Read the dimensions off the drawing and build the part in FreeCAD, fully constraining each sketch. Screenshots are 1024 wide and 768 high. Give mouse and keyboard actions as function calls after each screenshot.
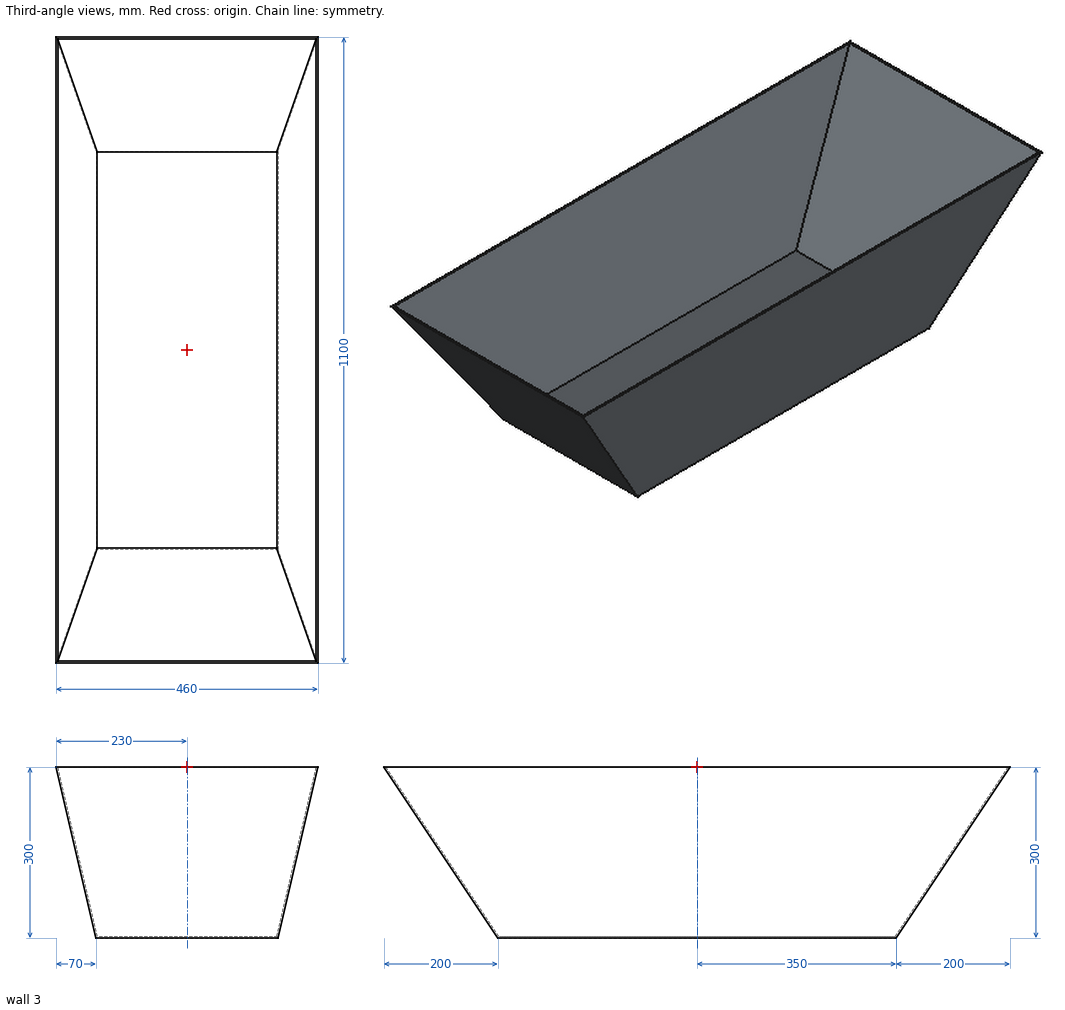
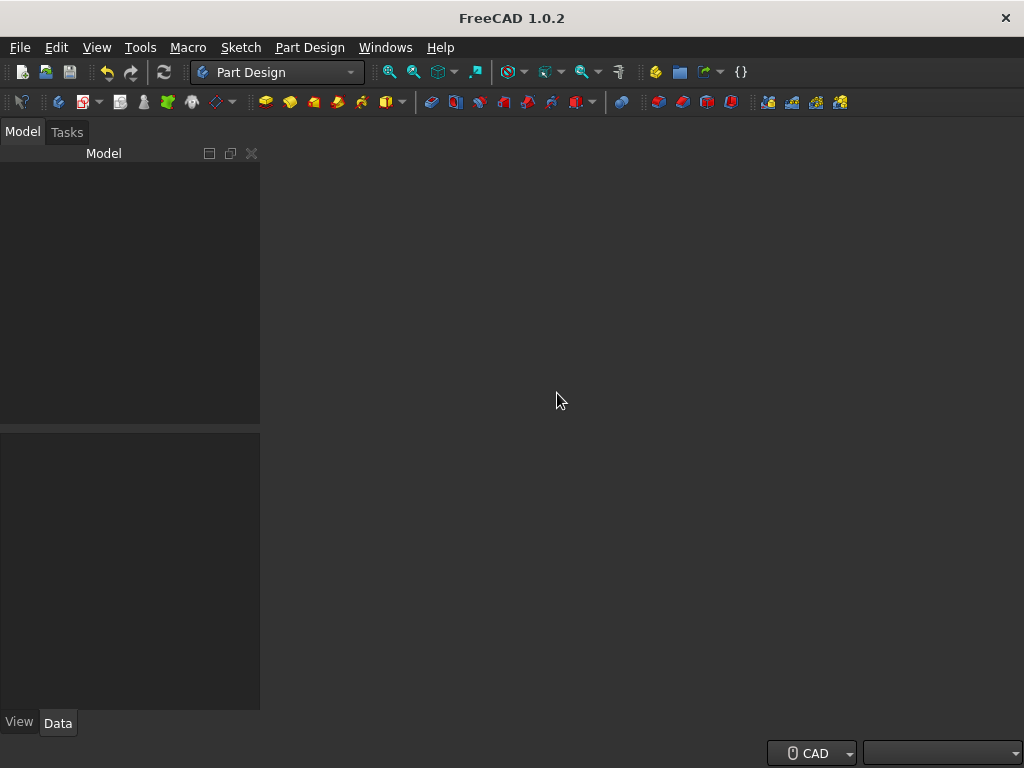
click(22, 72)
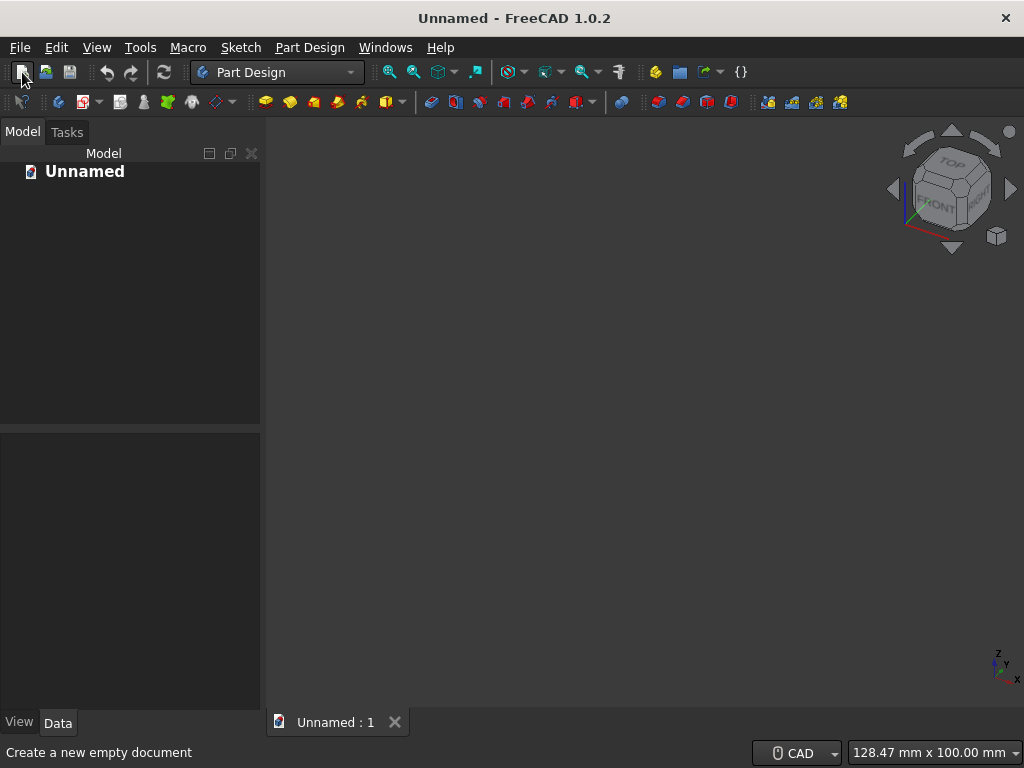
click(84, 102)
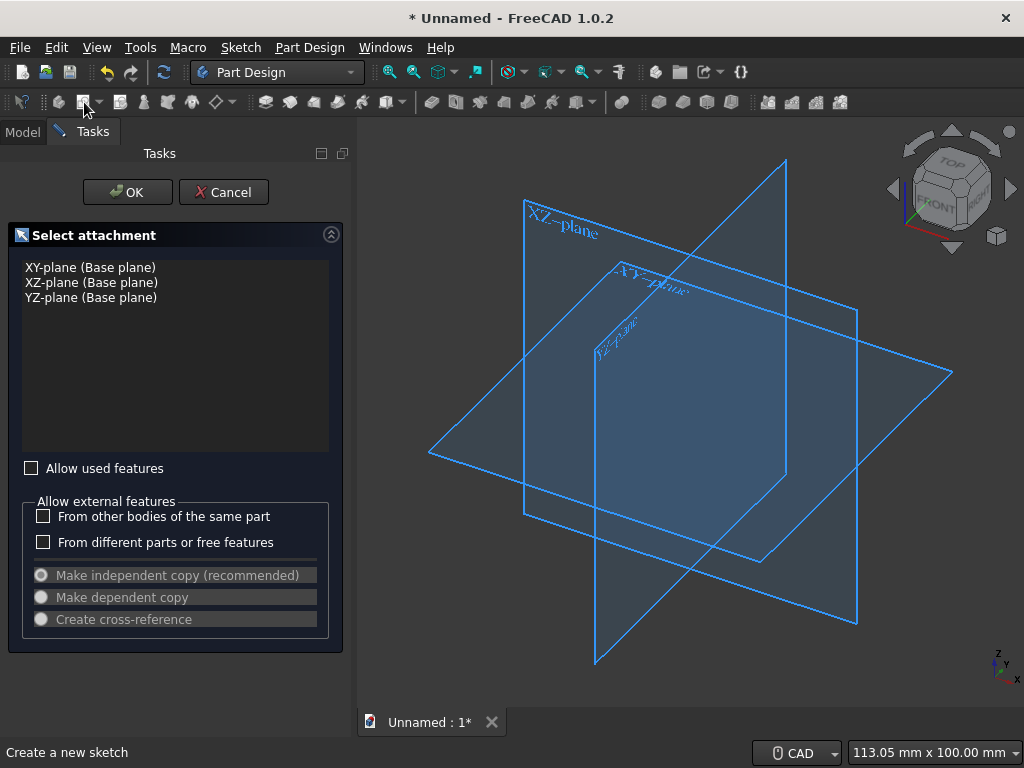
click(82, 268)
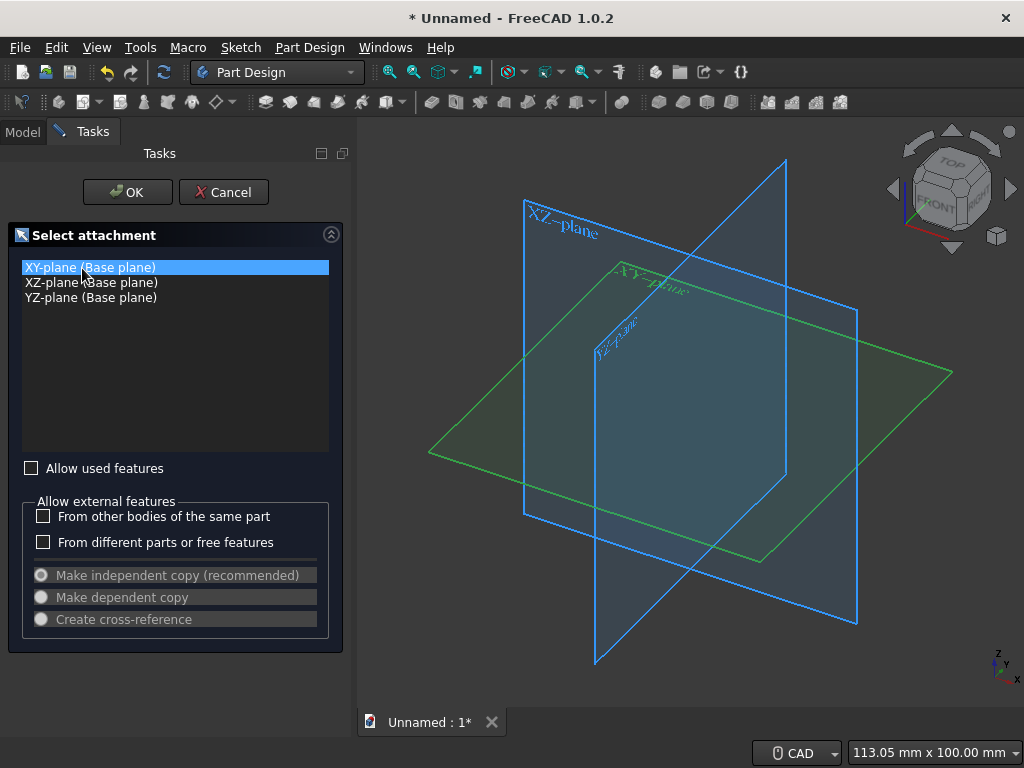
click(128, 192)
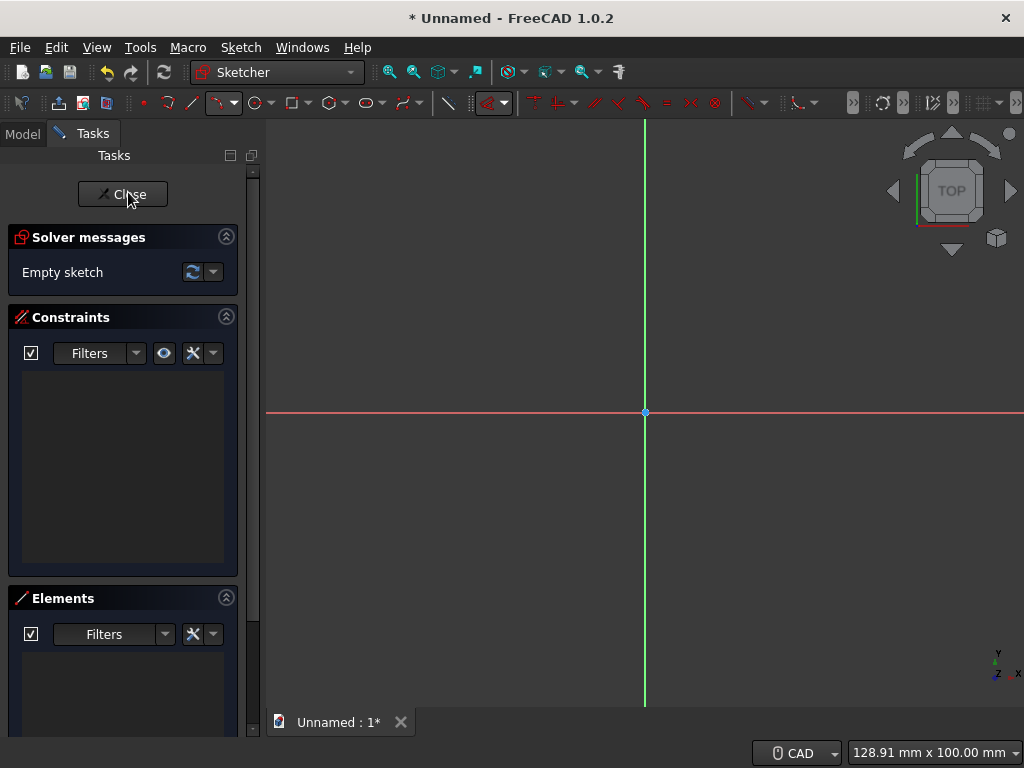
scroll(572, 413, down, 14)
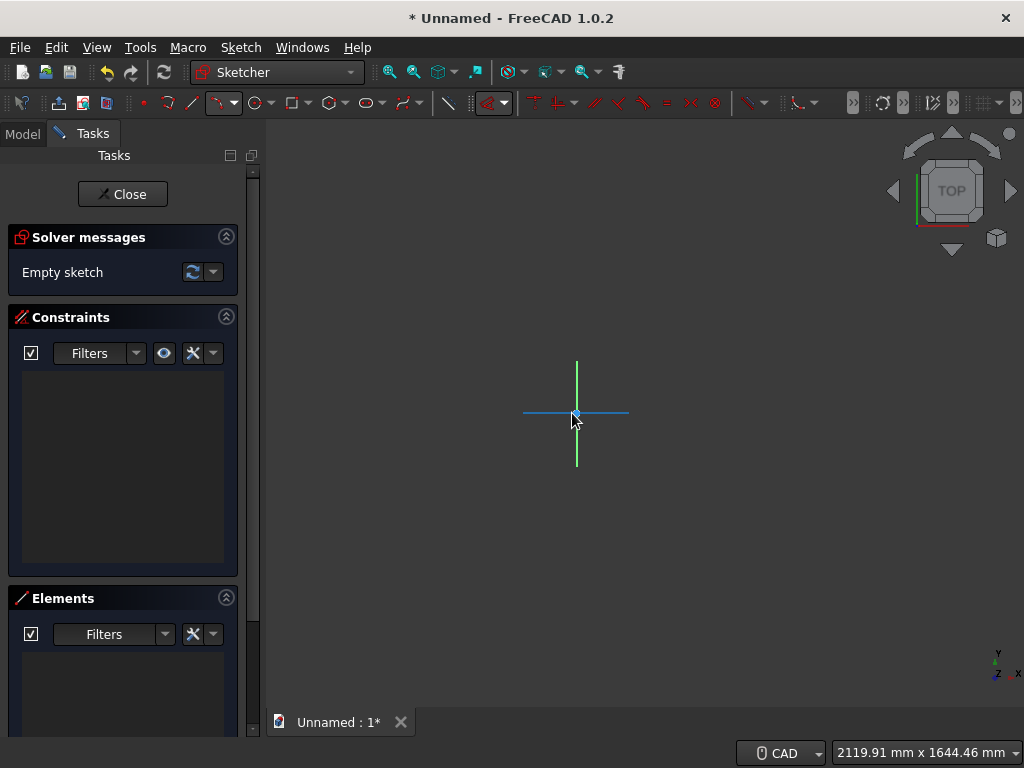
key(g)
key(v)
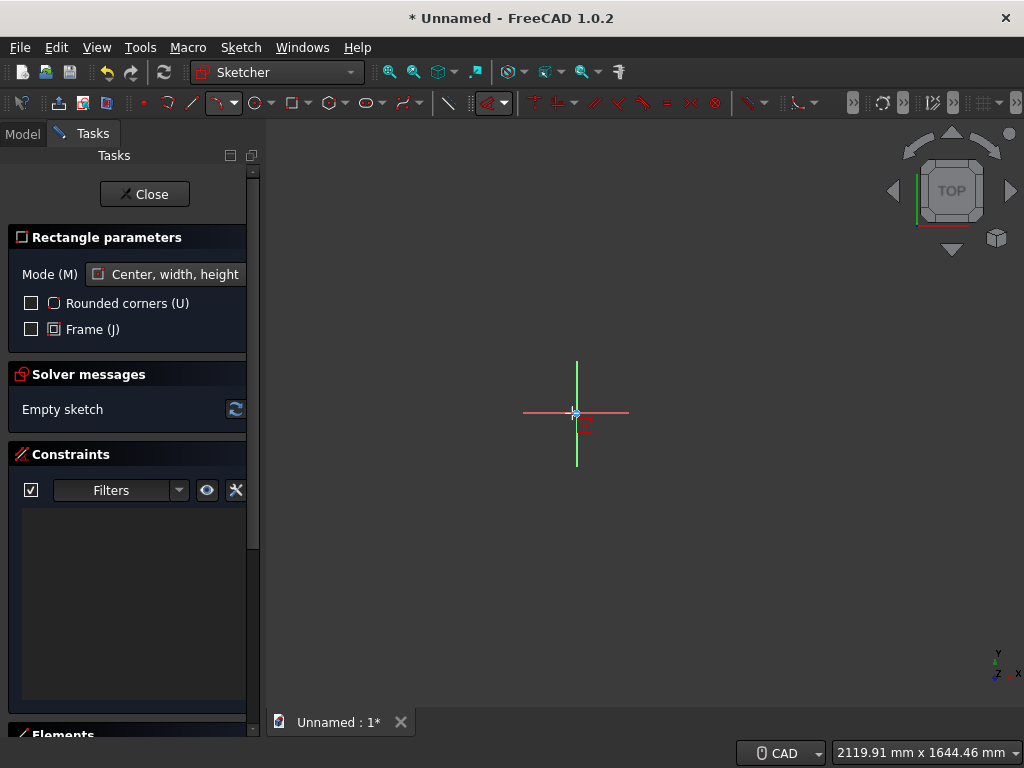
click(577, 413)
move(659, 217)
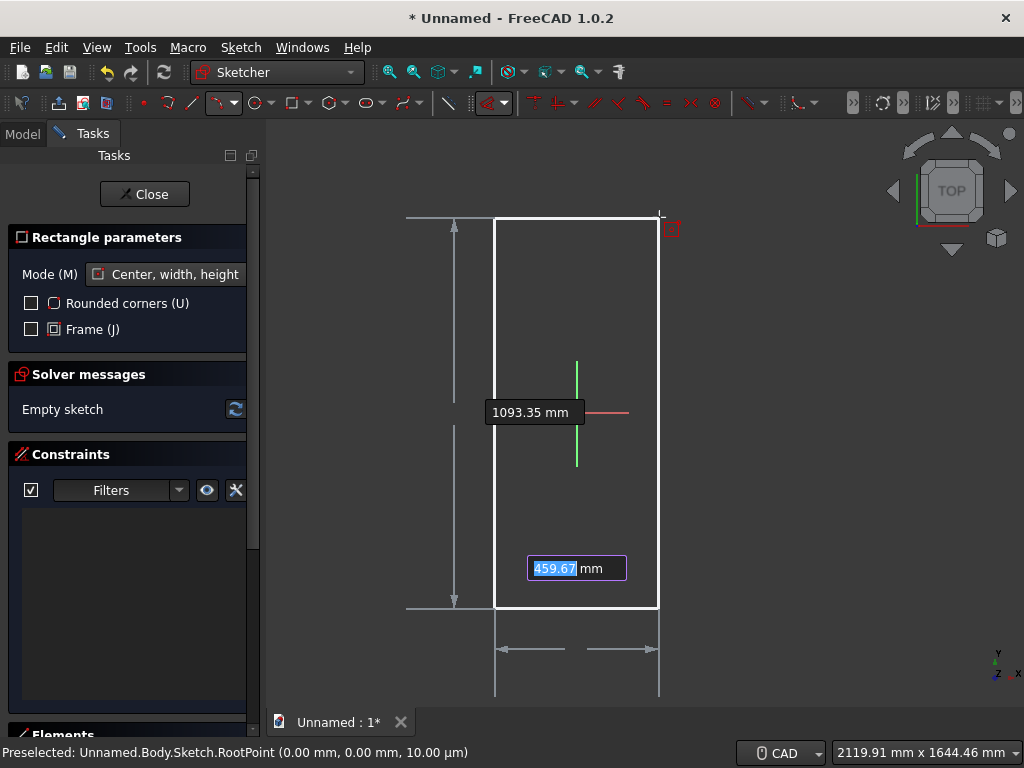
text(460)
key(Tab)
text(1100)
key(Return)
key(Escape)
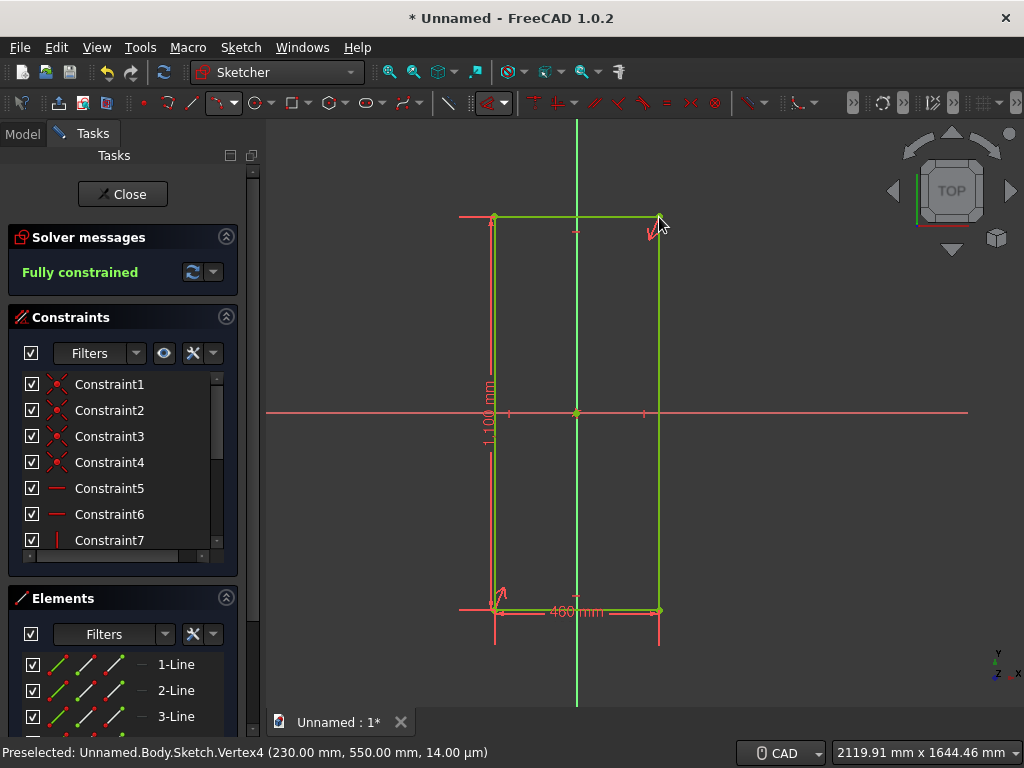
click(123, 194)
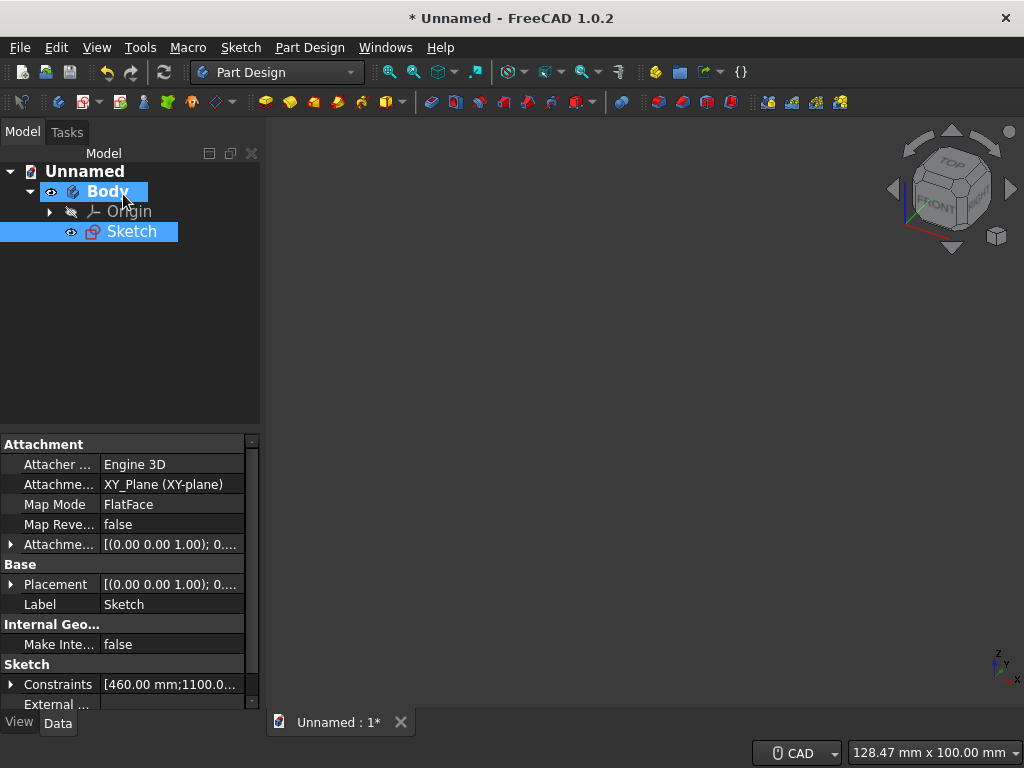
click(266, 102)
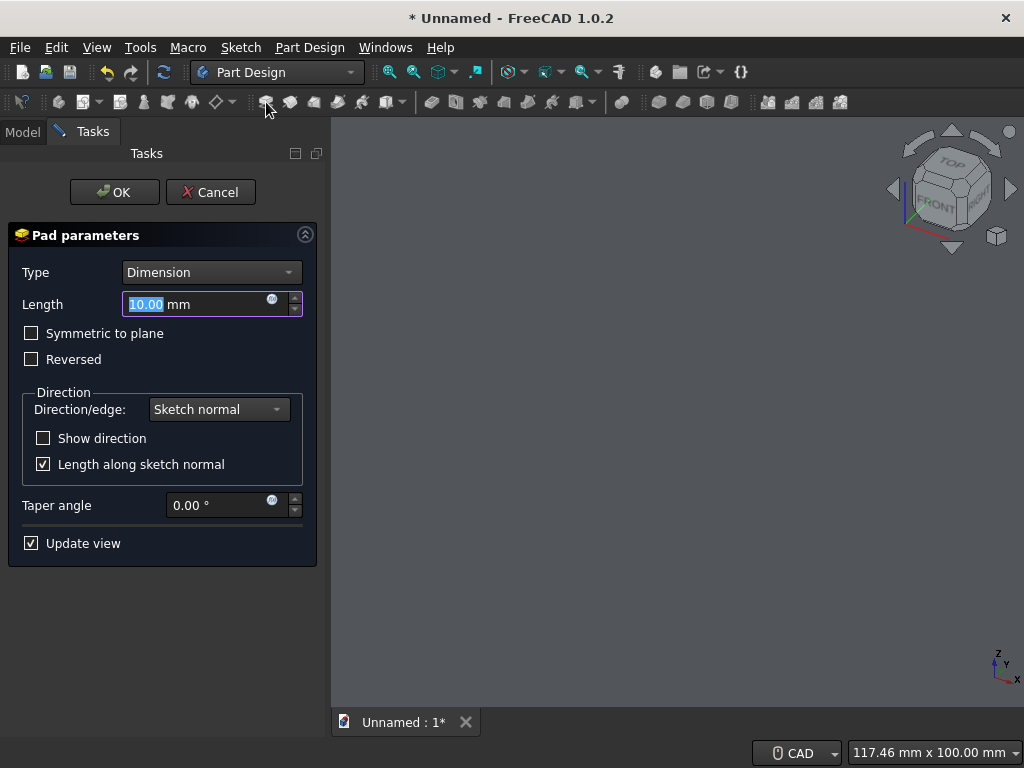
text(300)
key(Tab)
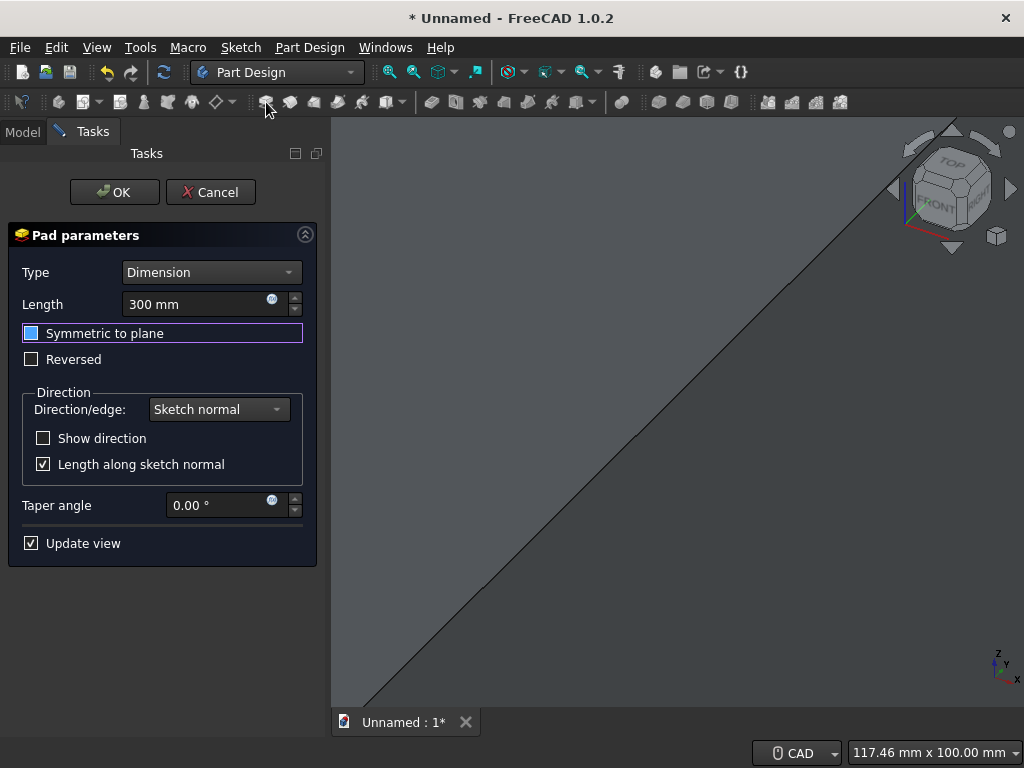
click(30, 359)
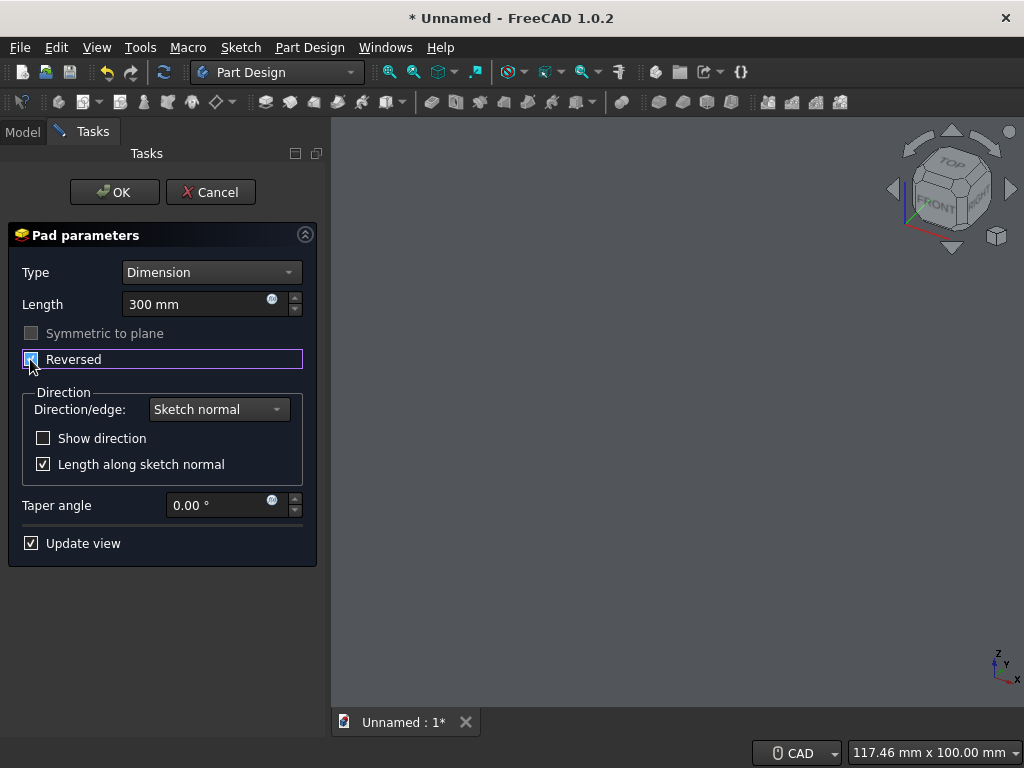
click(115, 192)